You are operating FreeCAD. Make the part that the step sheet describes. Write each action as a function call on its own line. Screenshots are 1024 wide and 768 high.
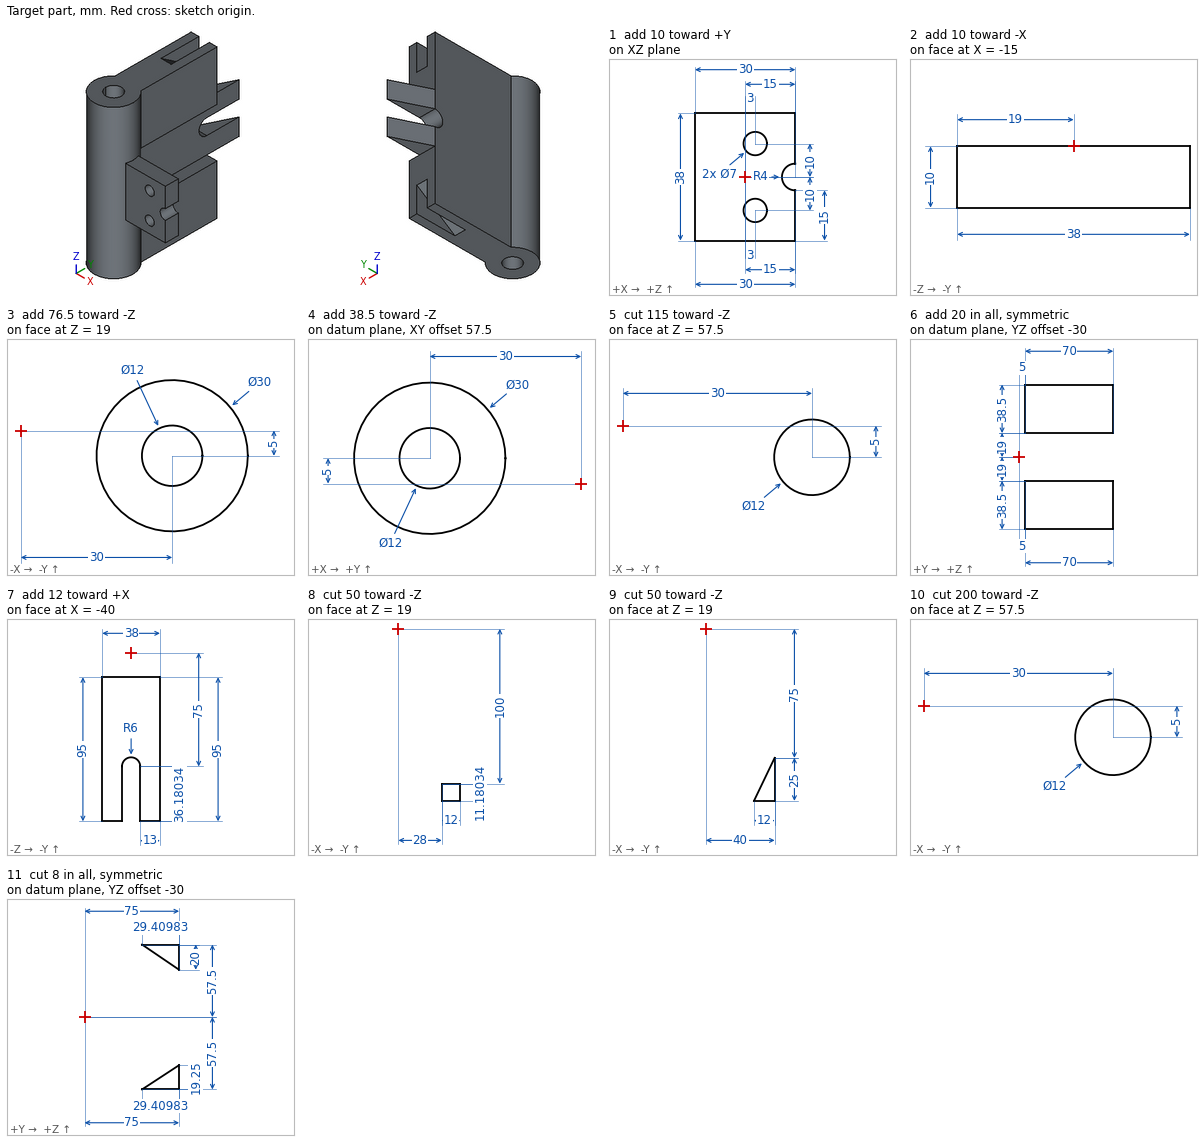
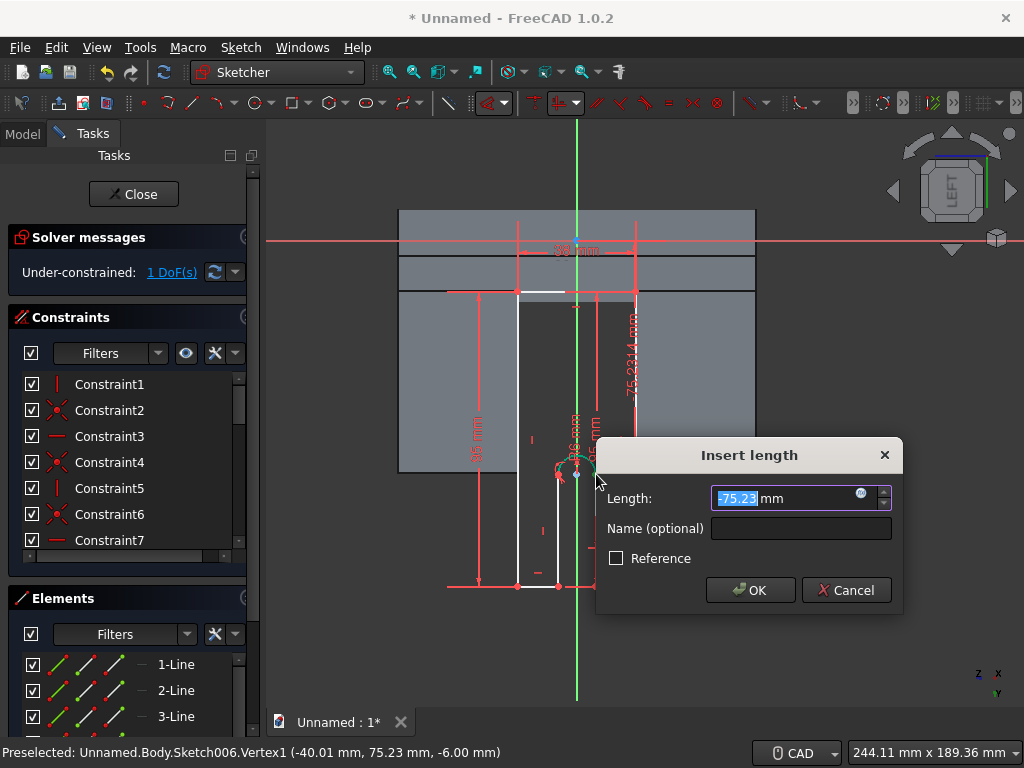
text(-75)
key(Return)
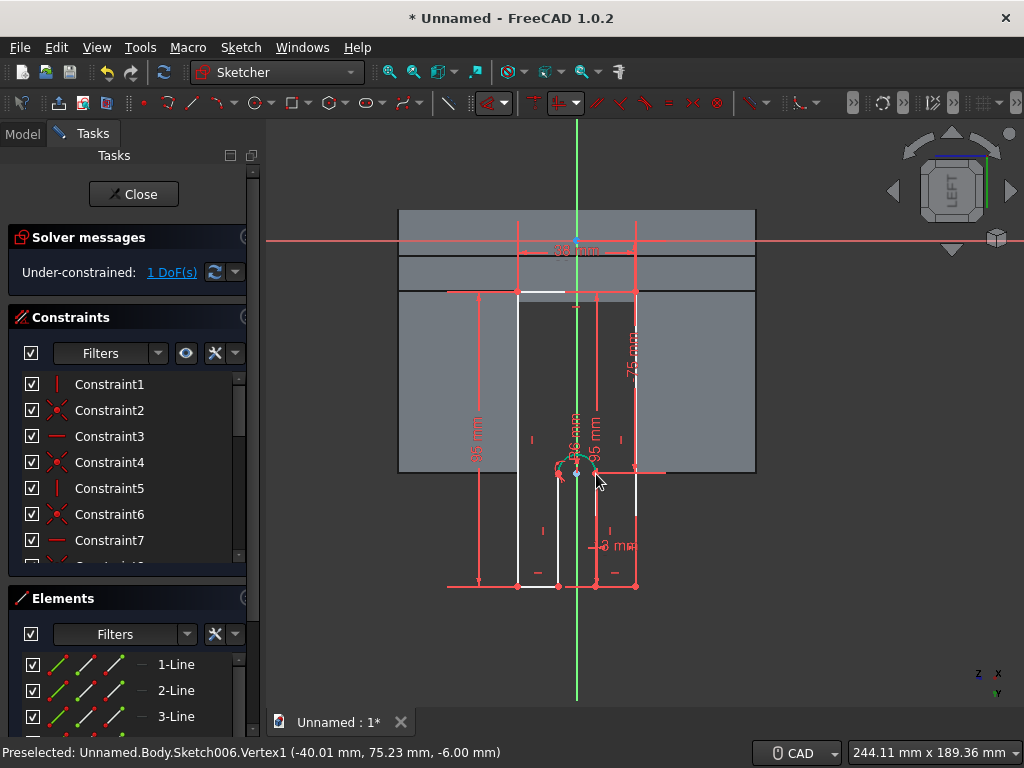
click(596, 507)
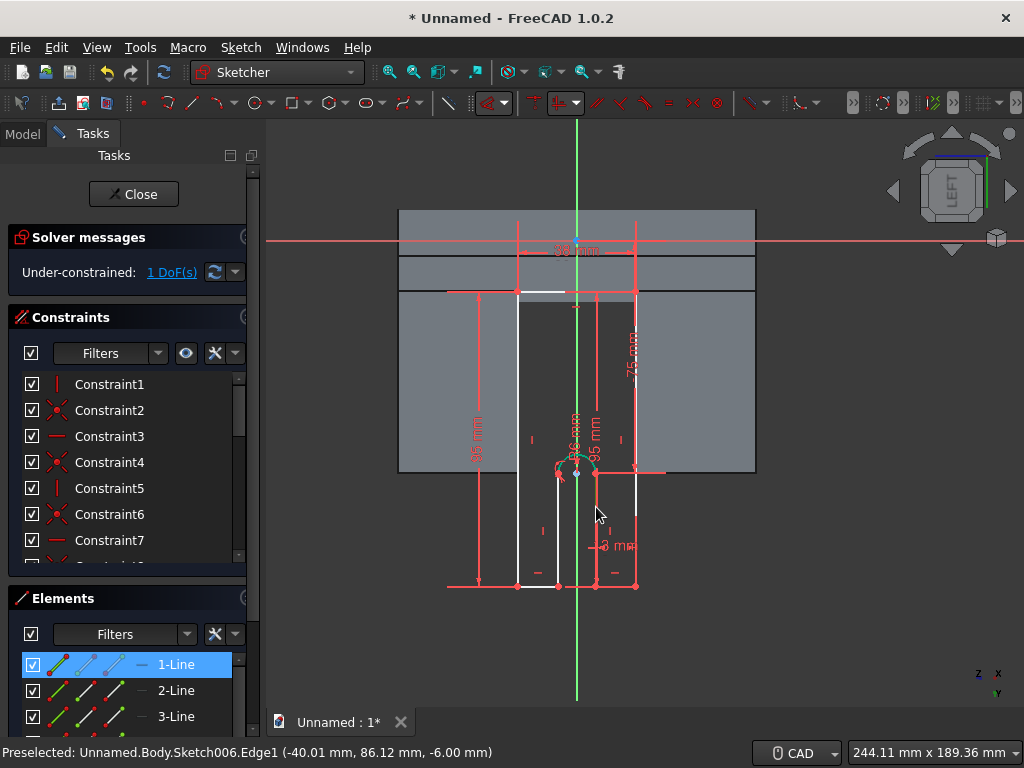
key(i)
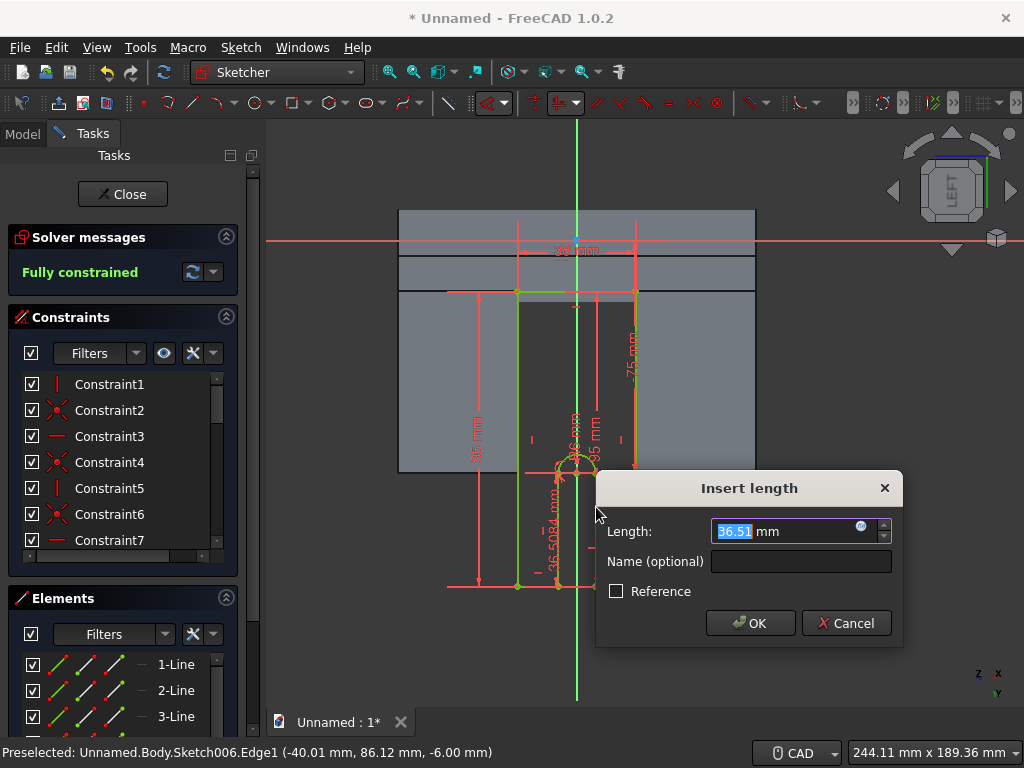
text(36.18034)
key(Return)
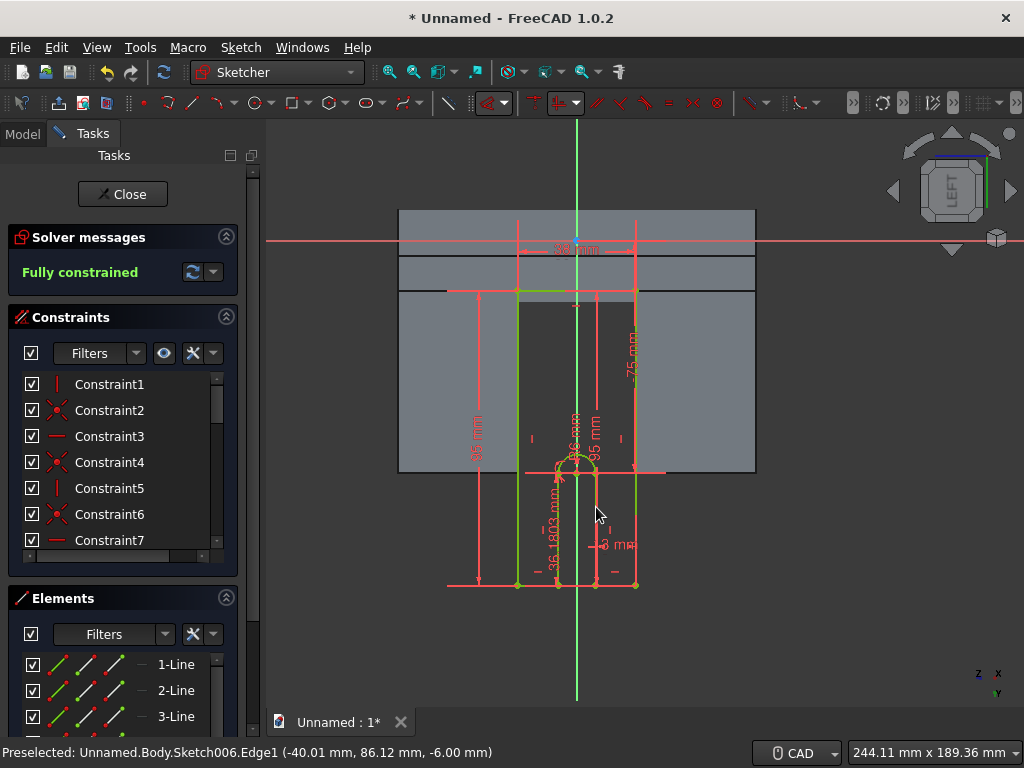
click(123, 194)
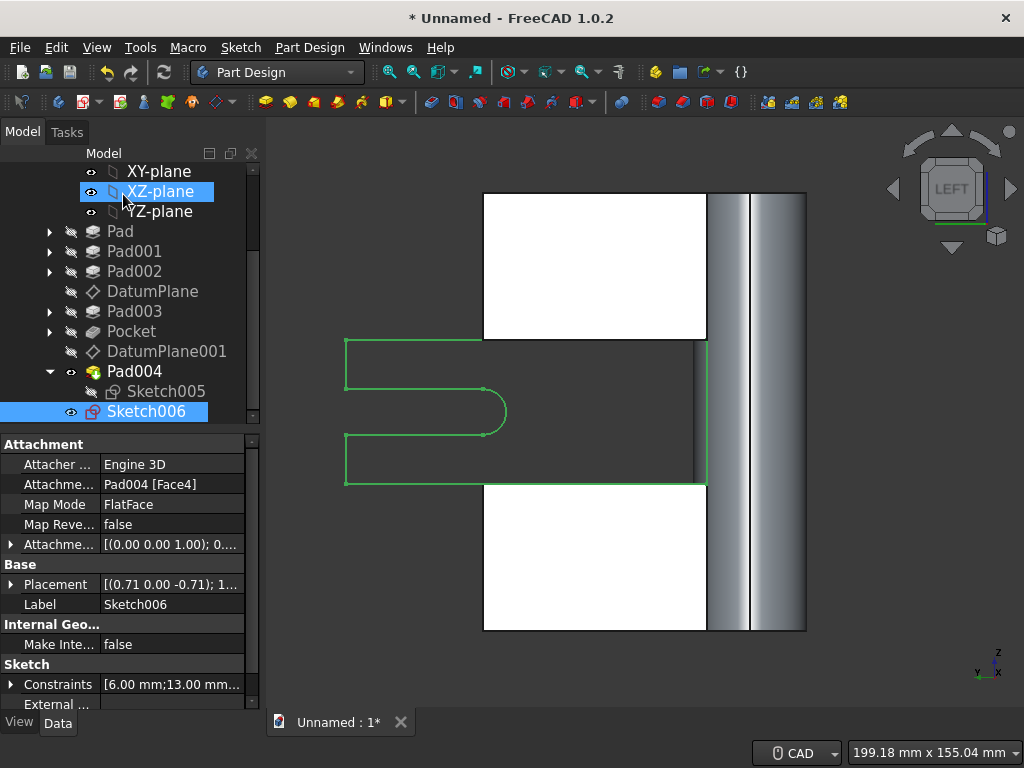
click(266, 102)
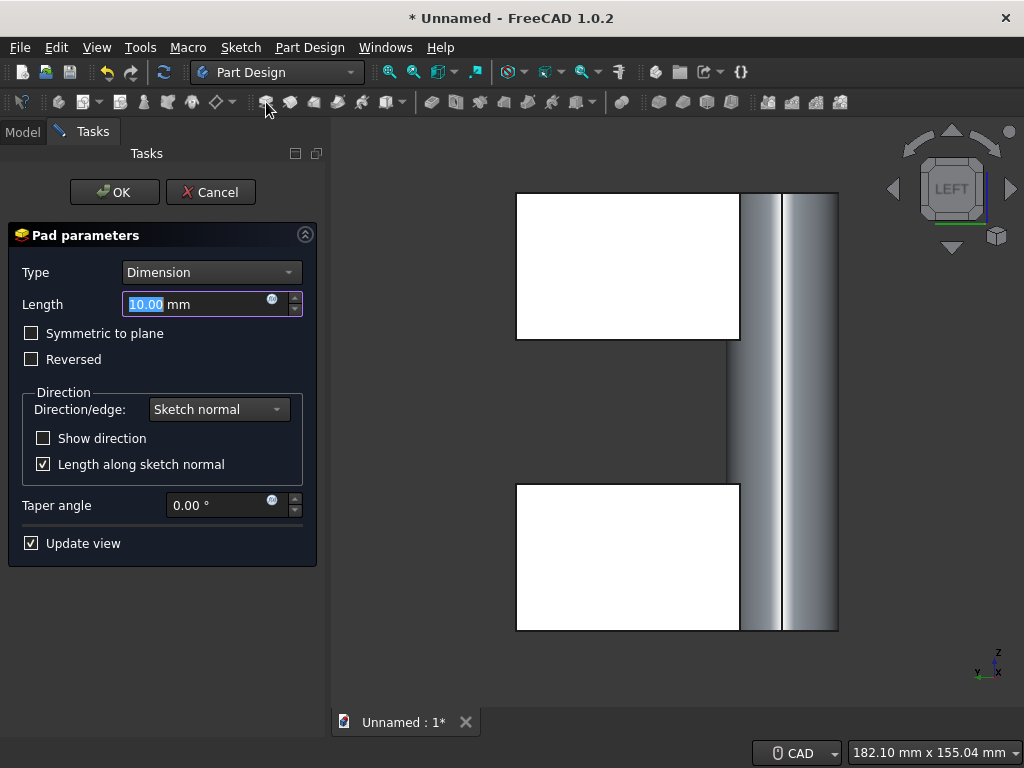
text(12)
key(Tab)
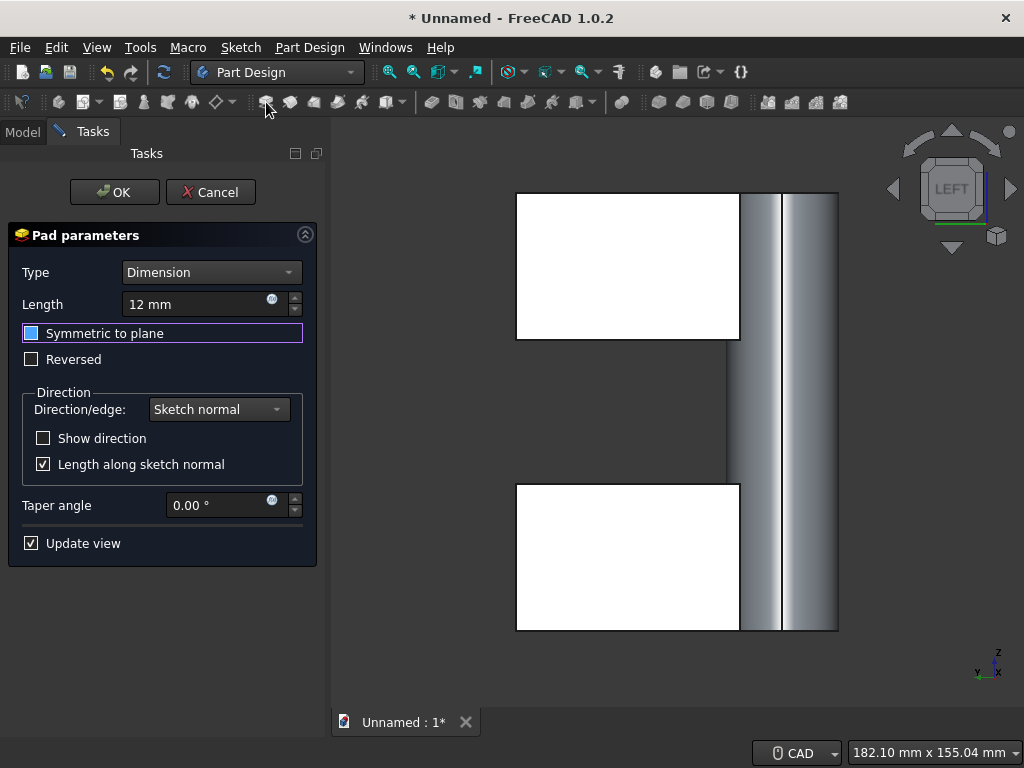
click(30, 359)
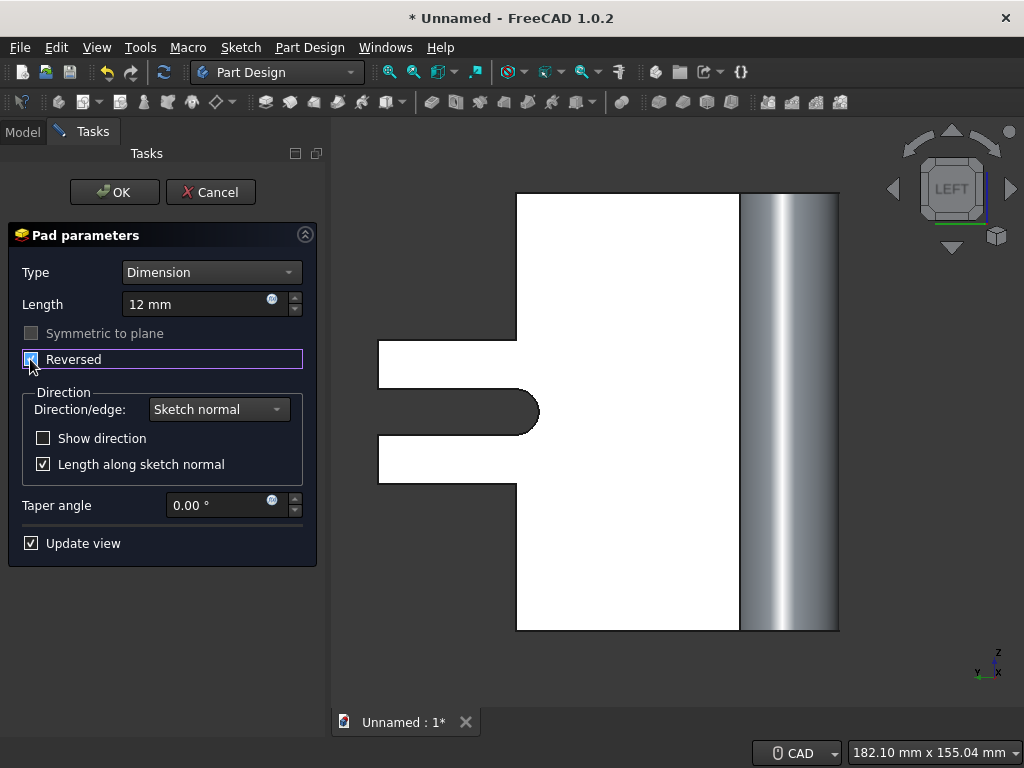
click(115, 192)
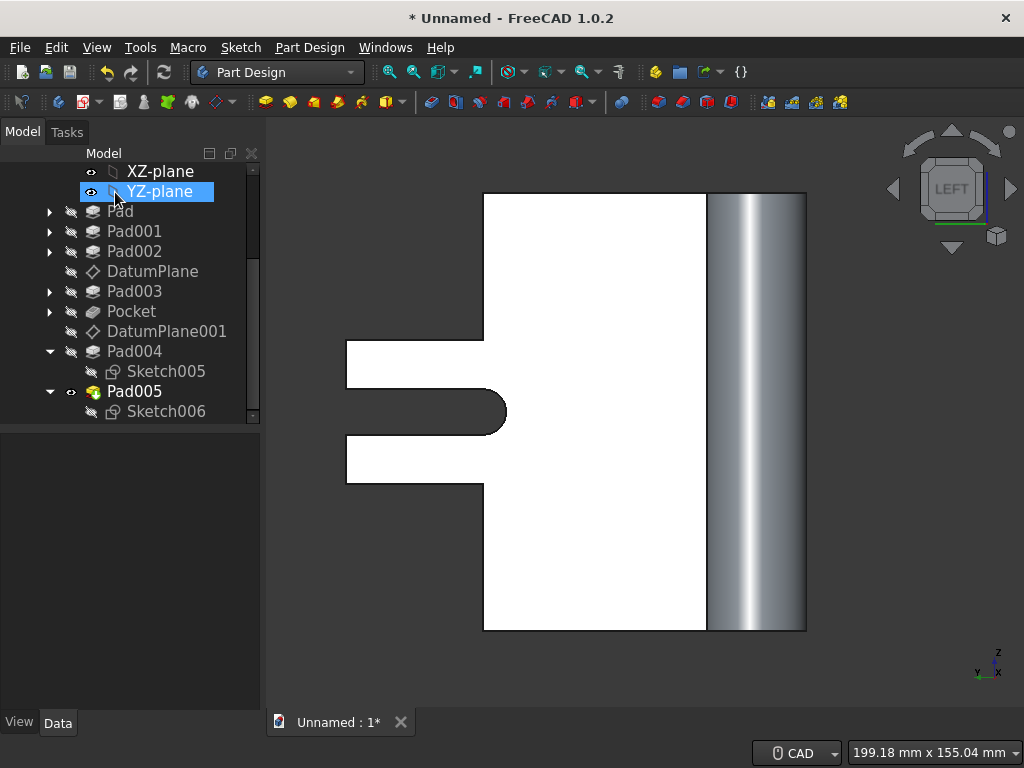
key(0)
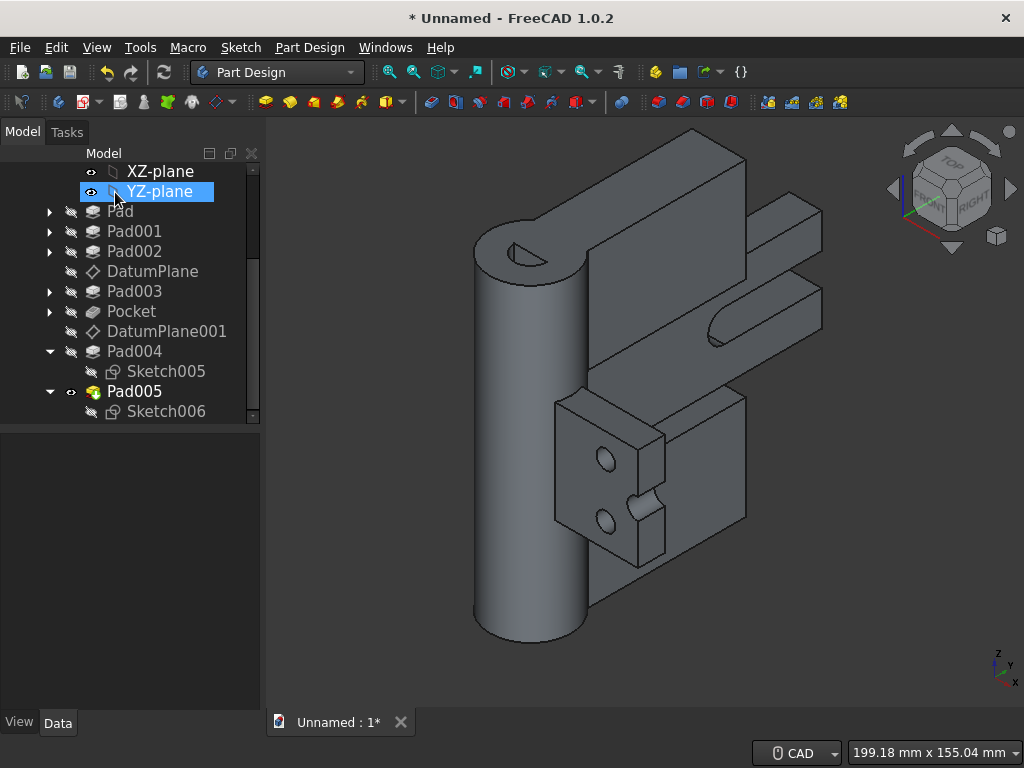
click(390, 72)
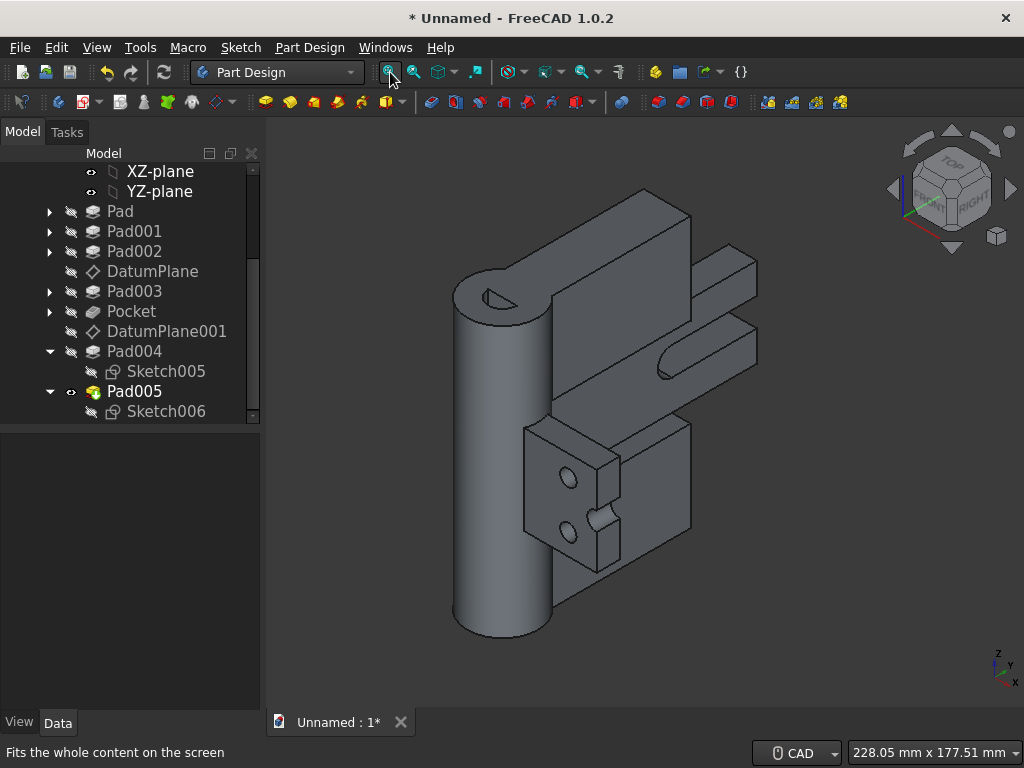
click(725, 262)